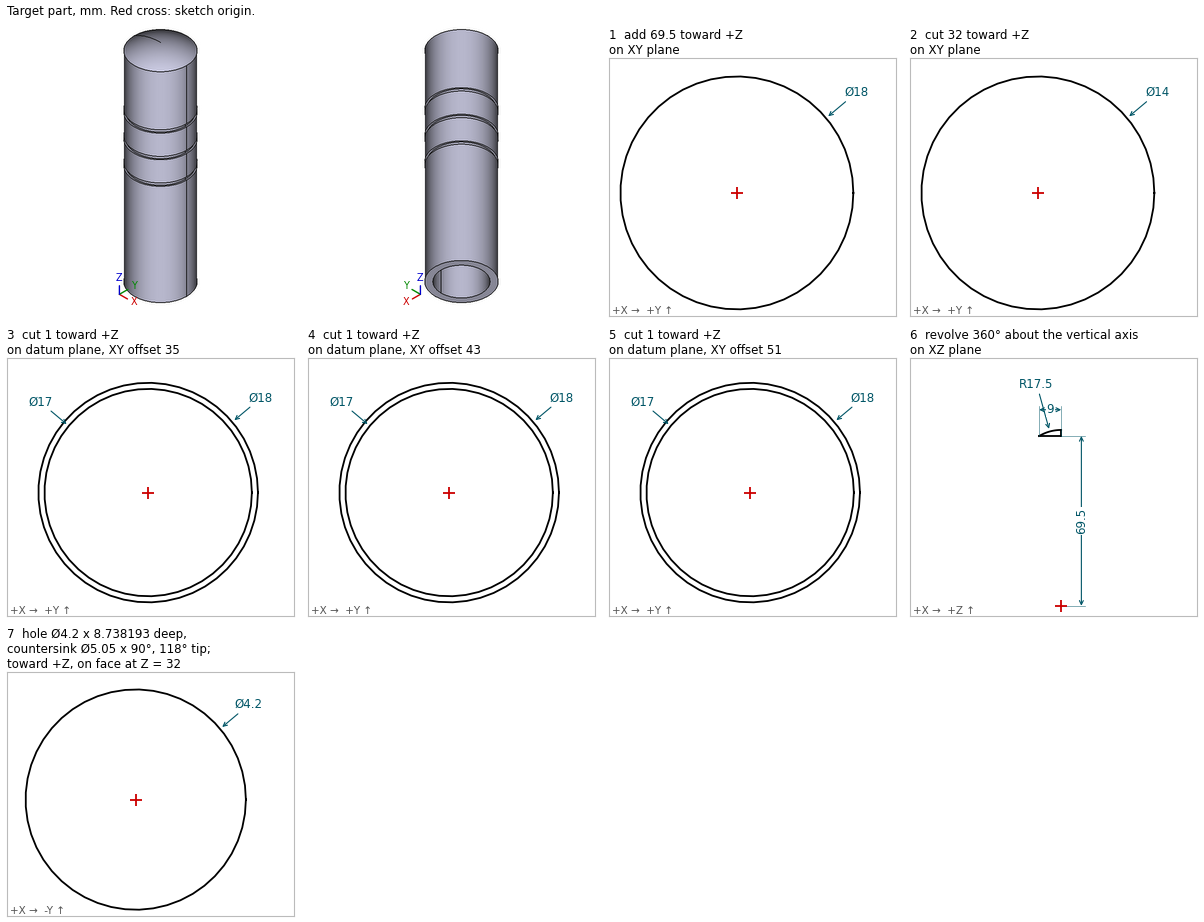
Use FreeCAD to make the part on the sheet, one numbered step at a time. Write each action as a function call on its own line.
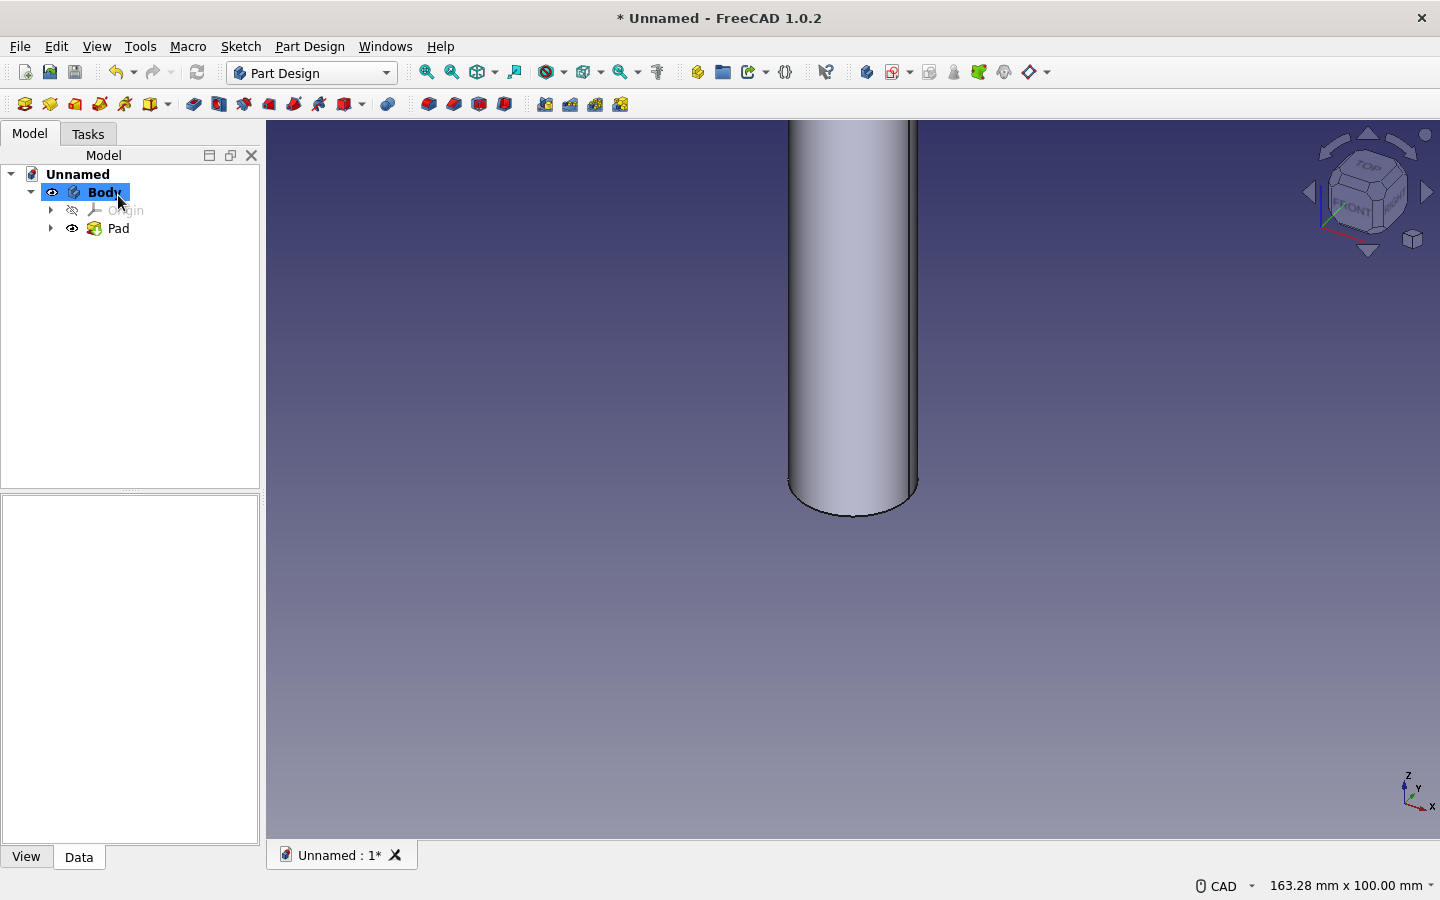
key(v)
key(f)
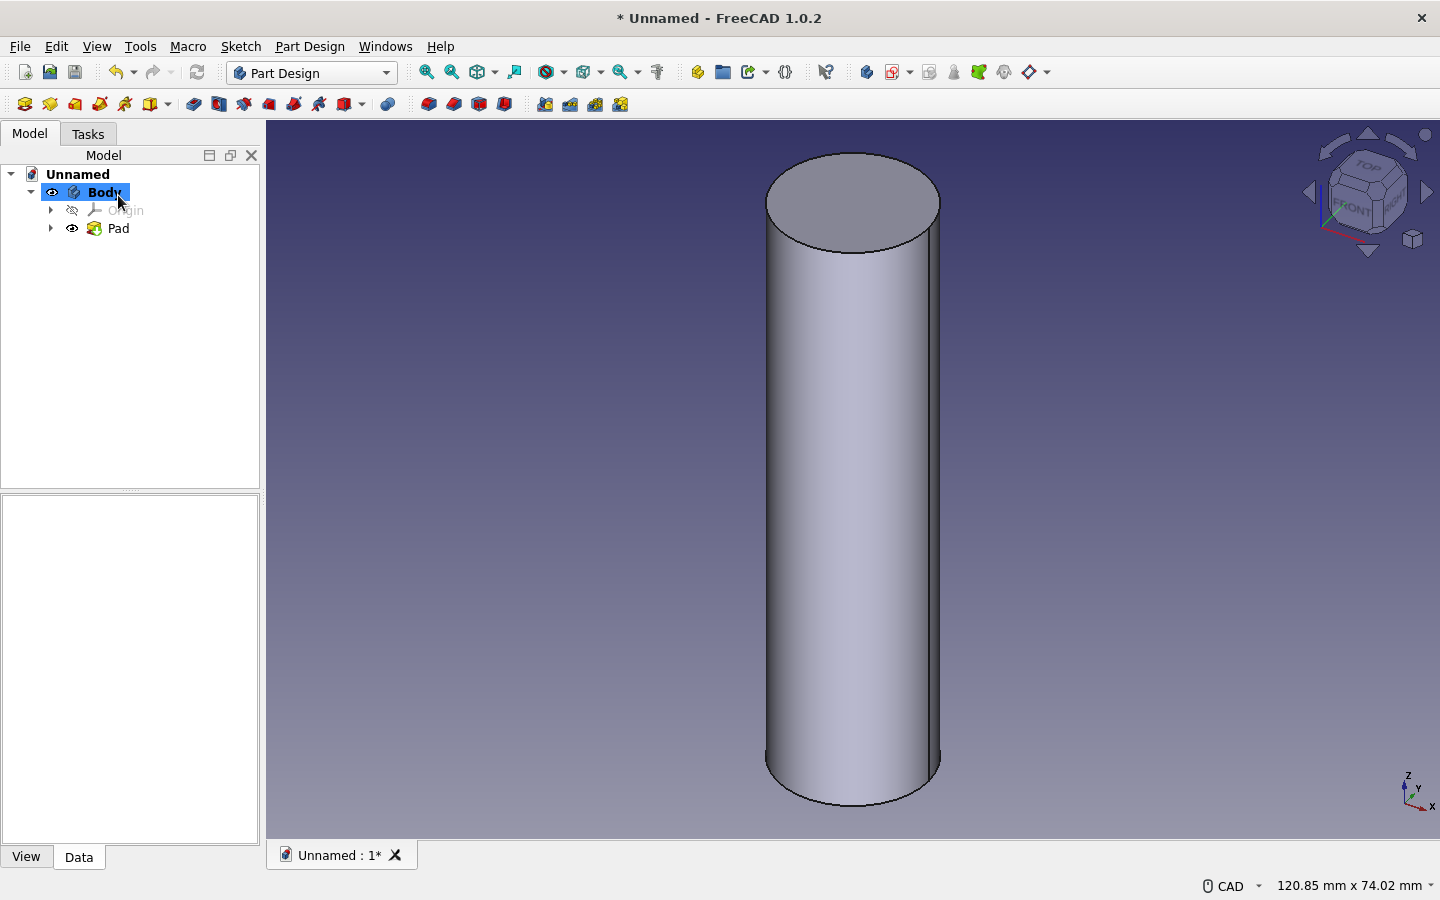
click(892, 72)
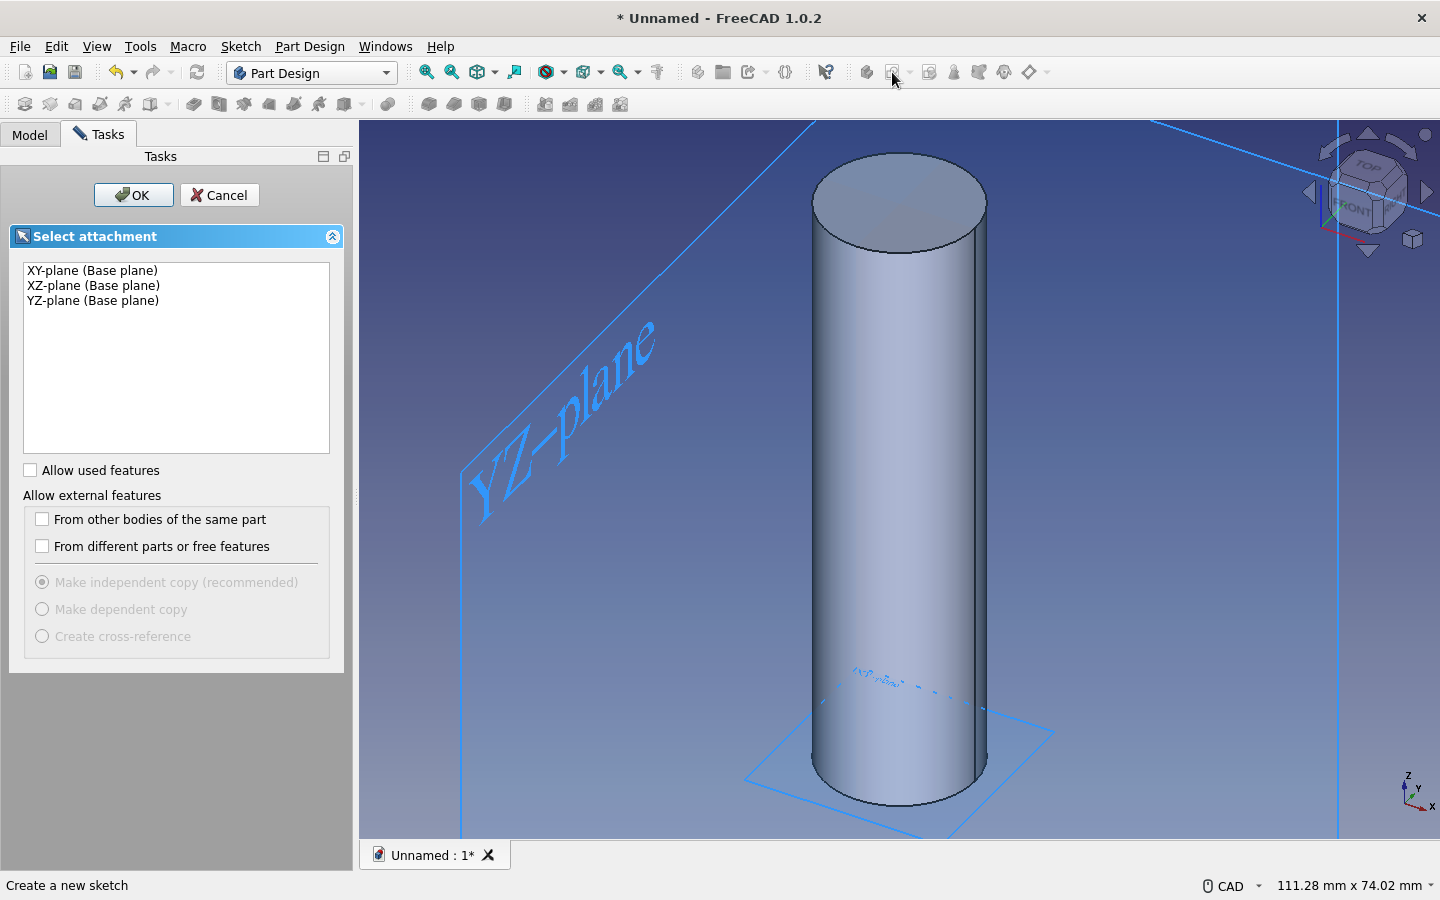
click(84, 270)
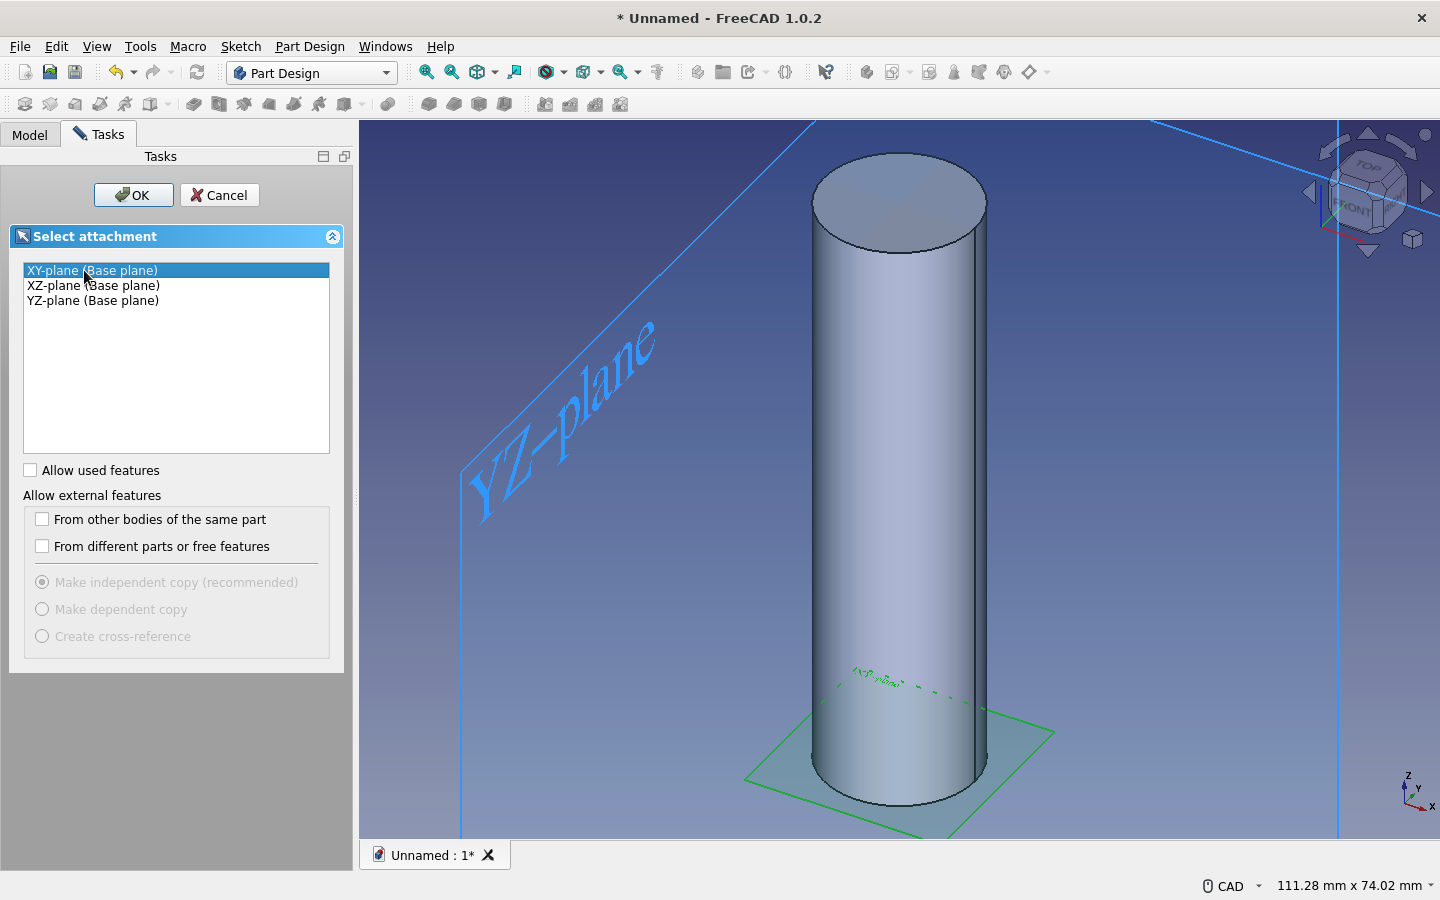
click(134, 195)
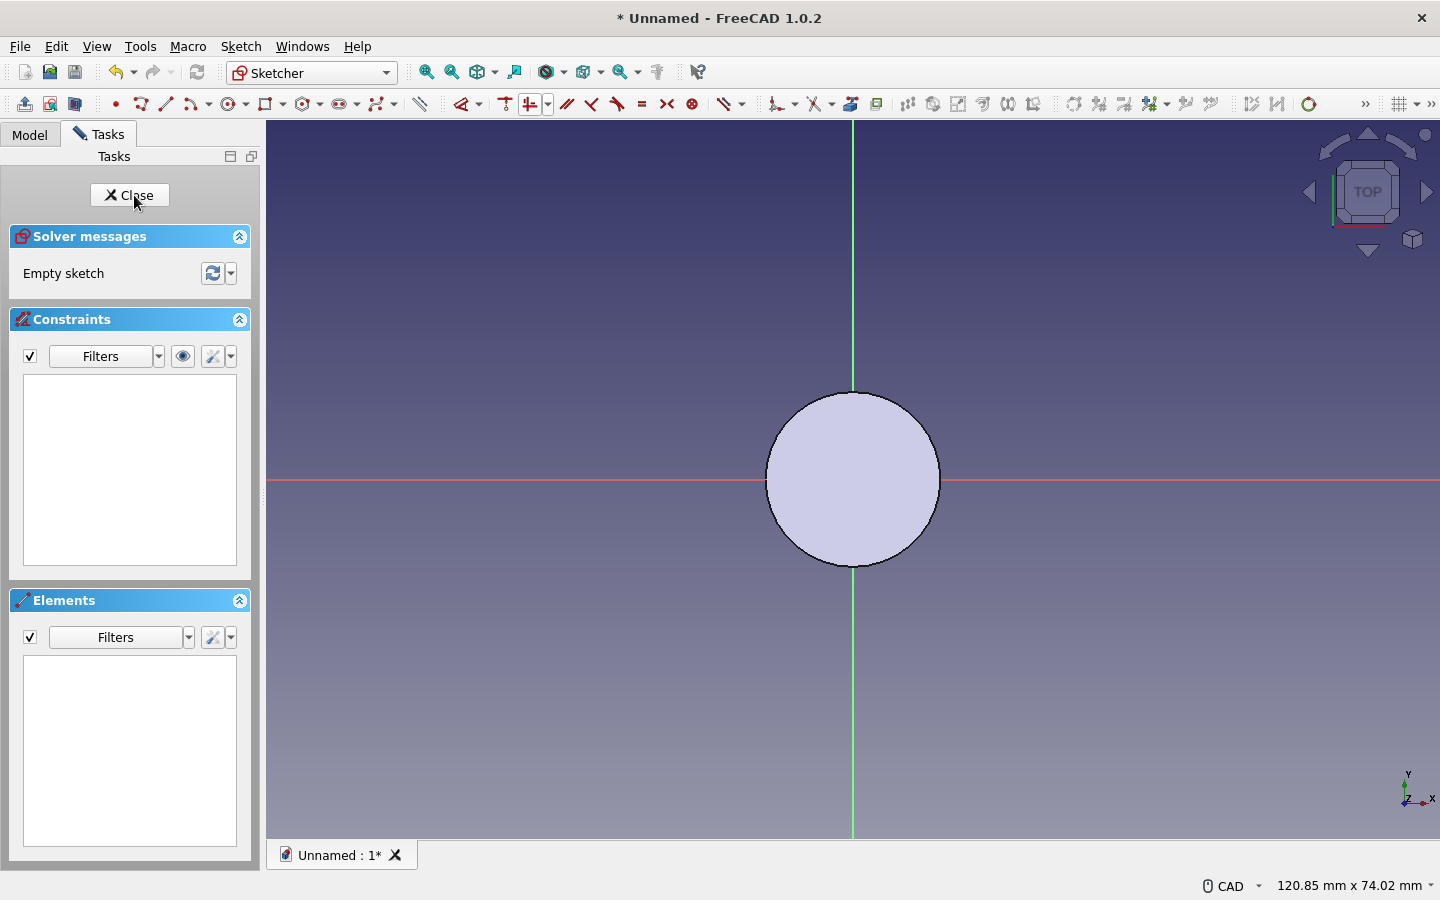
key(q)
key(s)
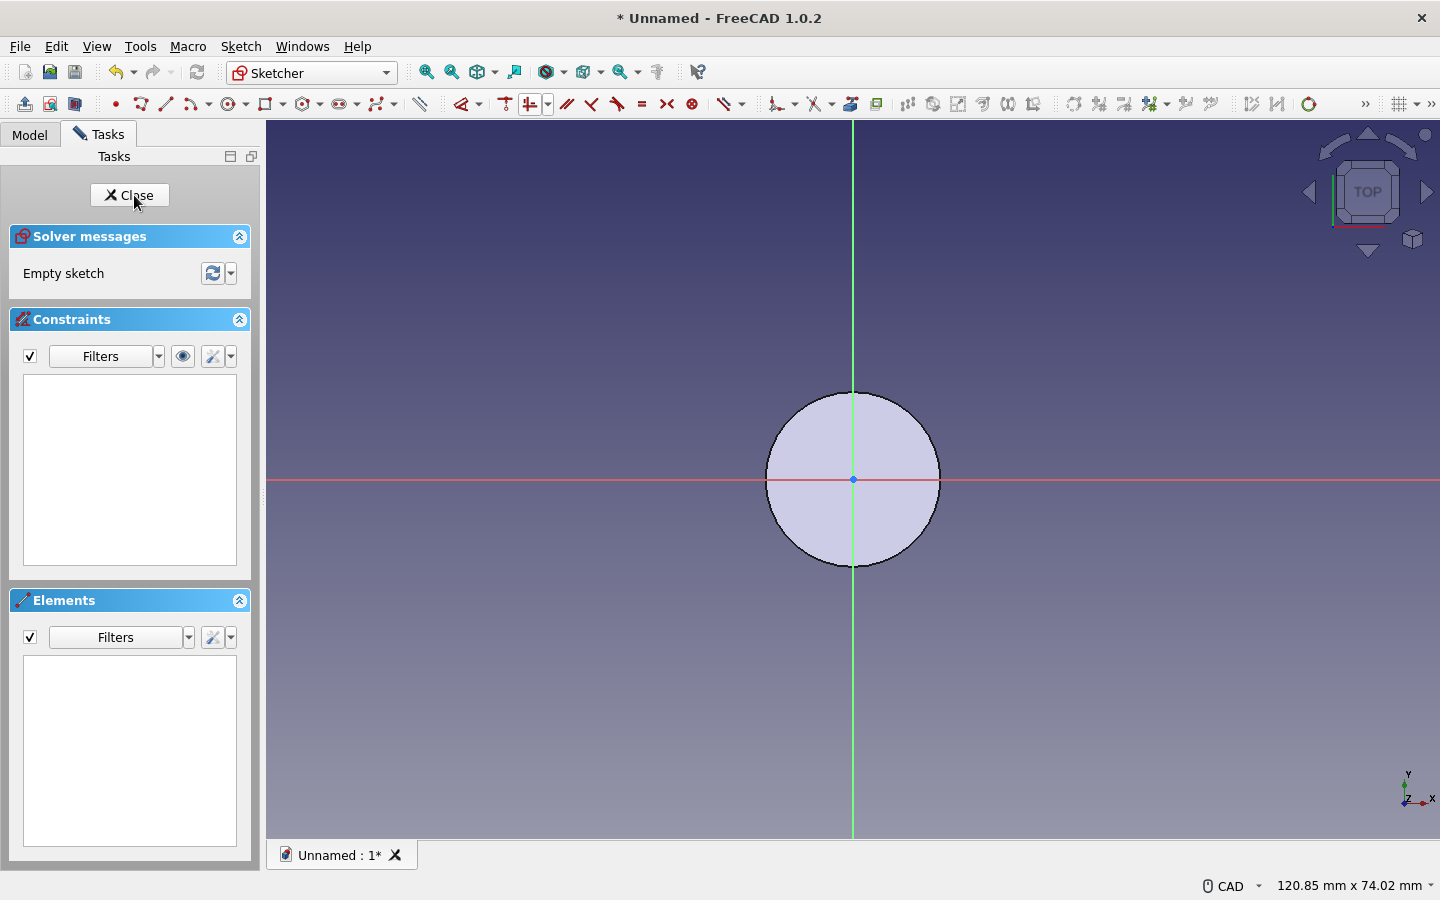
scroll(883, 480, up, 6)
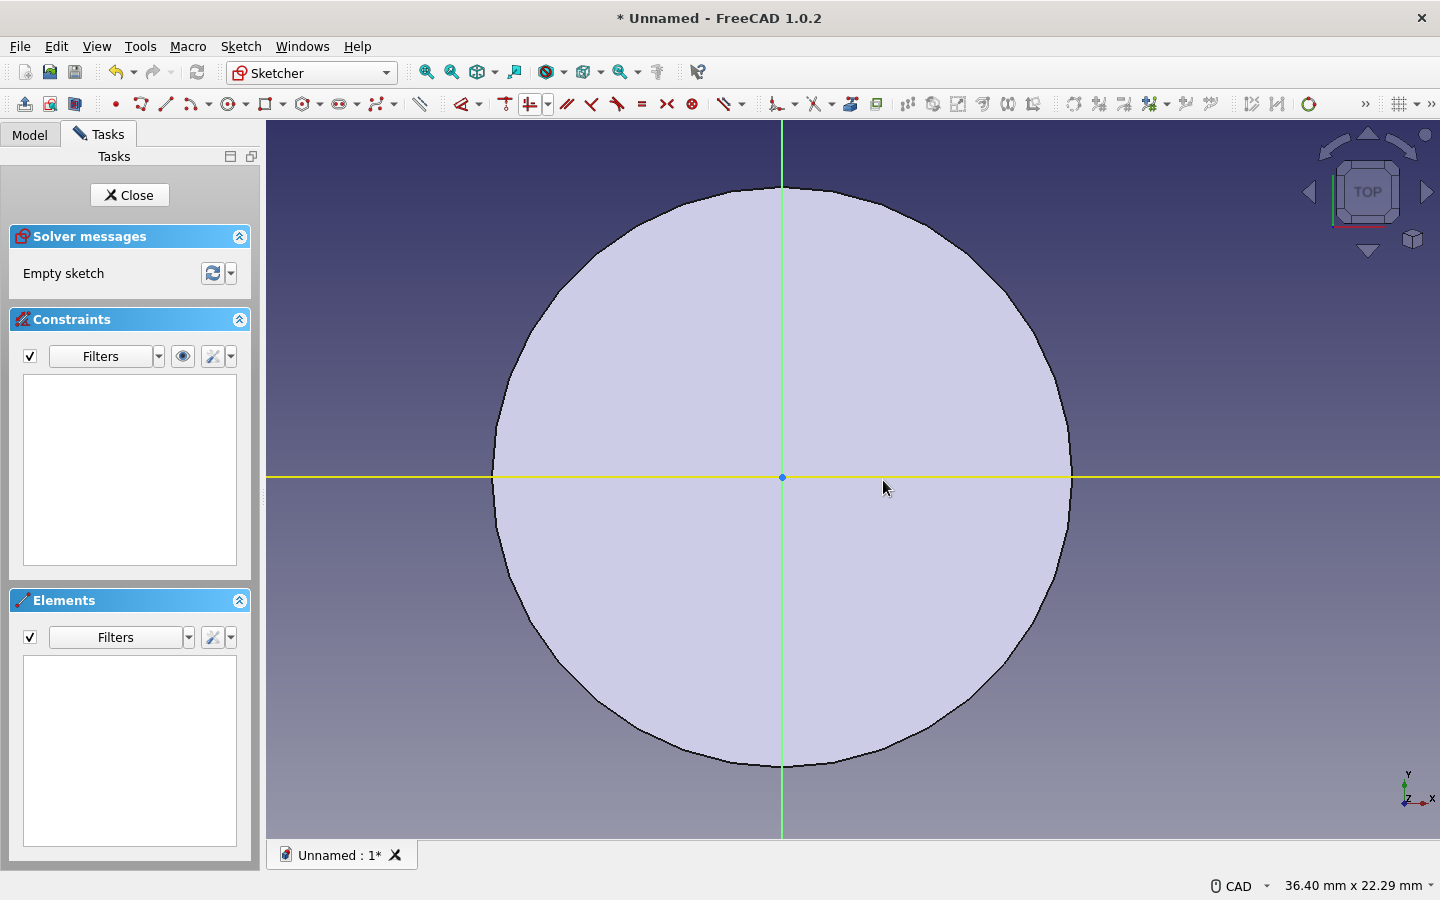
key(g)
key(c)